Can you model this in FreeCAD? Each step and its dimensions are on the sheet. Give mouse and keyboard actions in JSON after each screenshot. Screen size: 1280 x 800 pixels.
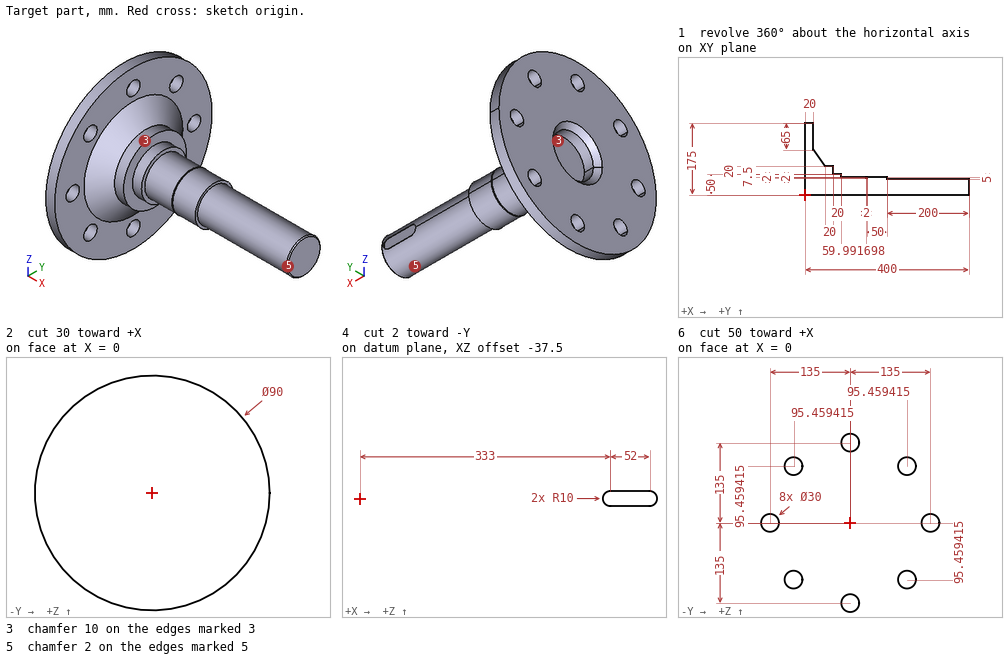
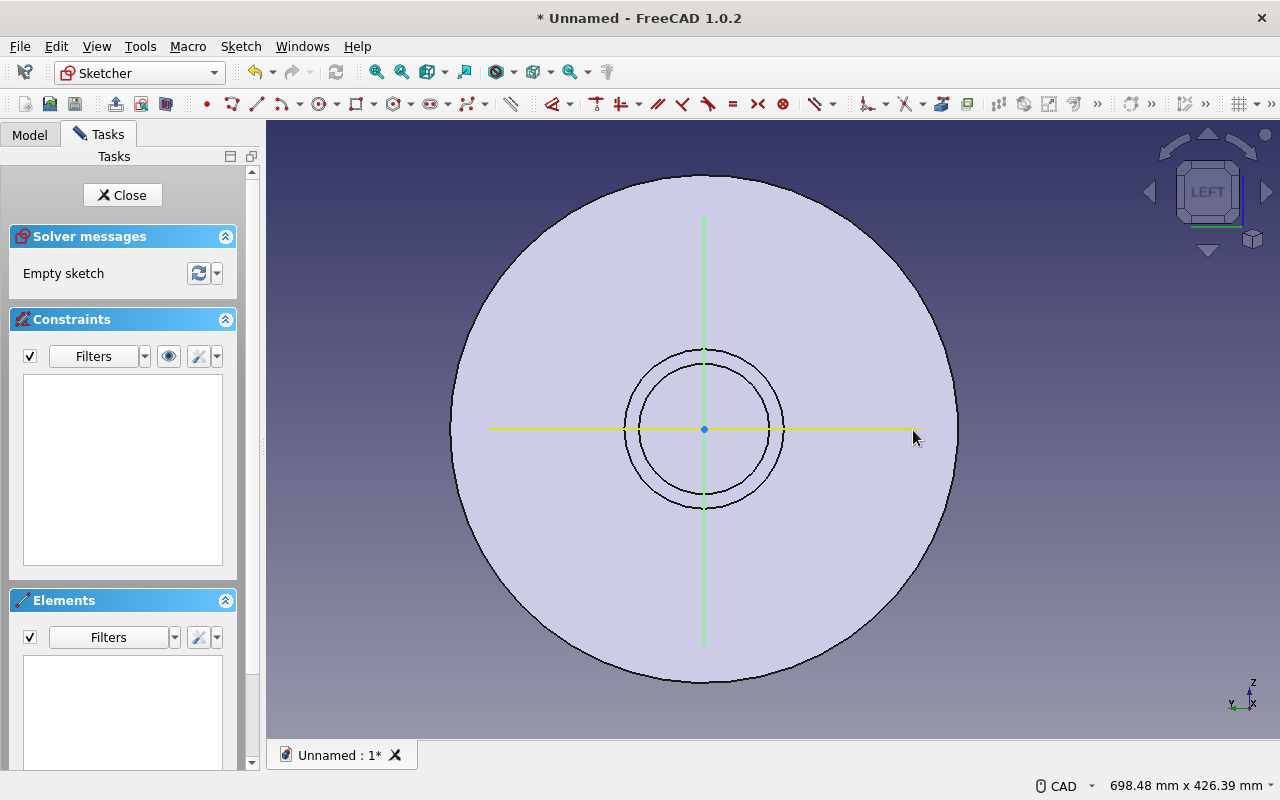
{"action": "left_click", "coordinate": [318, 104]}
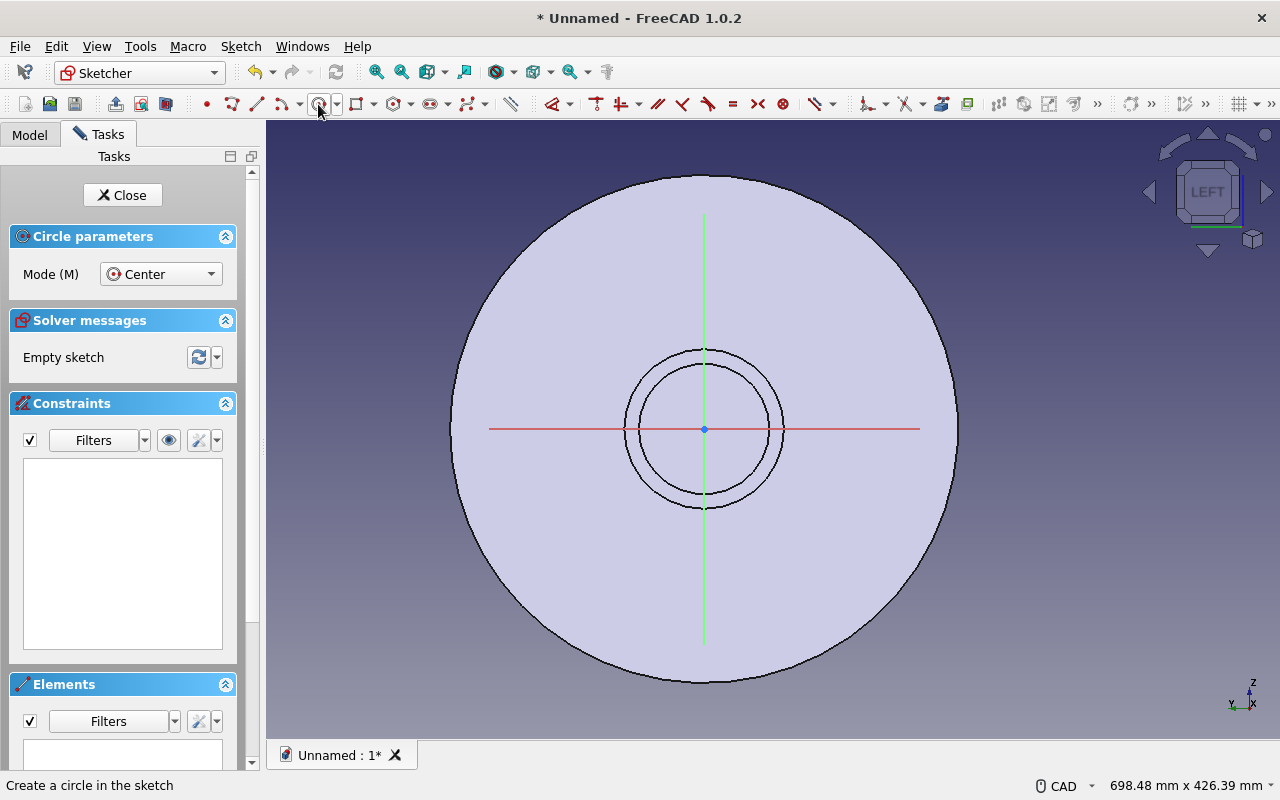
{"action": "left_click", "coordinate": [508, 429]}
{"action": "mouse_move", "coordinate": [524, 414]}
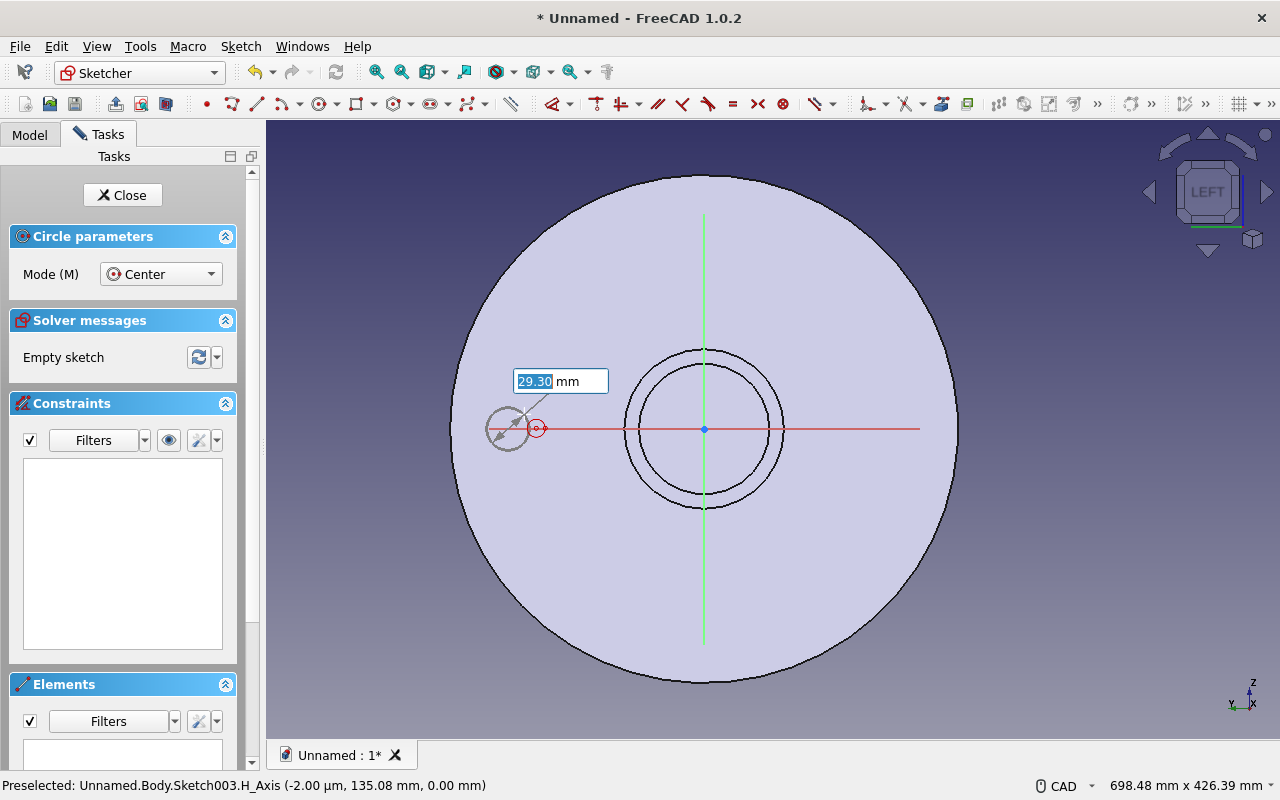
{"action": "type", "text": "30"}
{"action": "key", "text": "Return"}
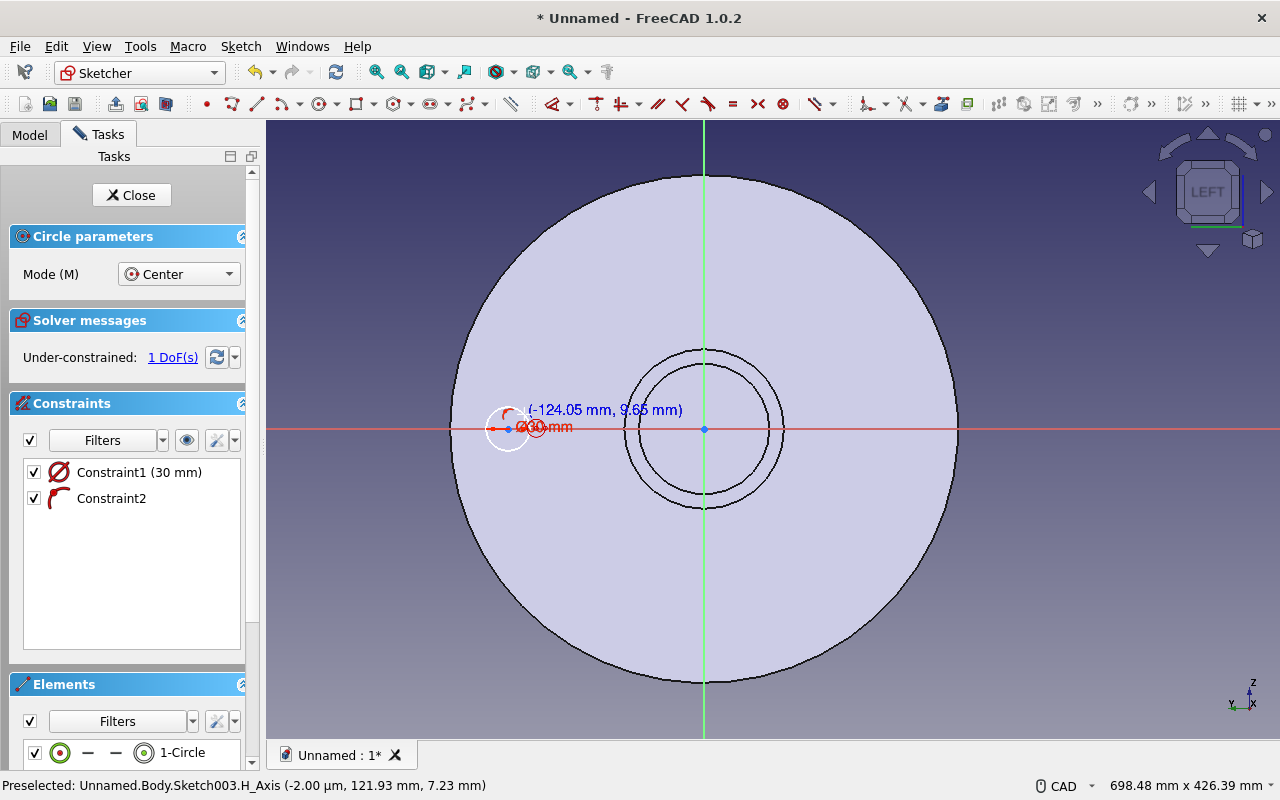
{"action": "left_click", "coordinate": [566, 290]}
{"action": "mouse_move", "coordinate": [581, 275]}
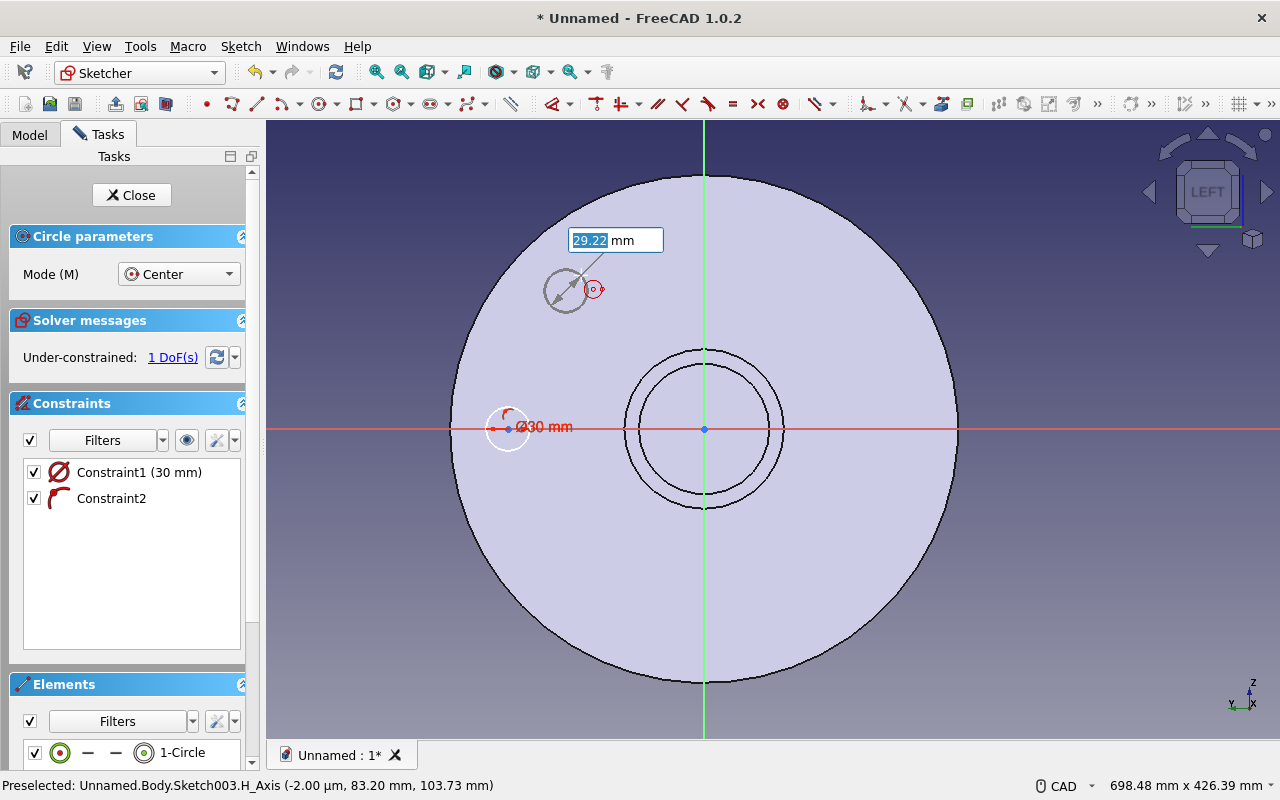
{"action": "type", "text": "30"}
{"action": "key", "text": "Return"}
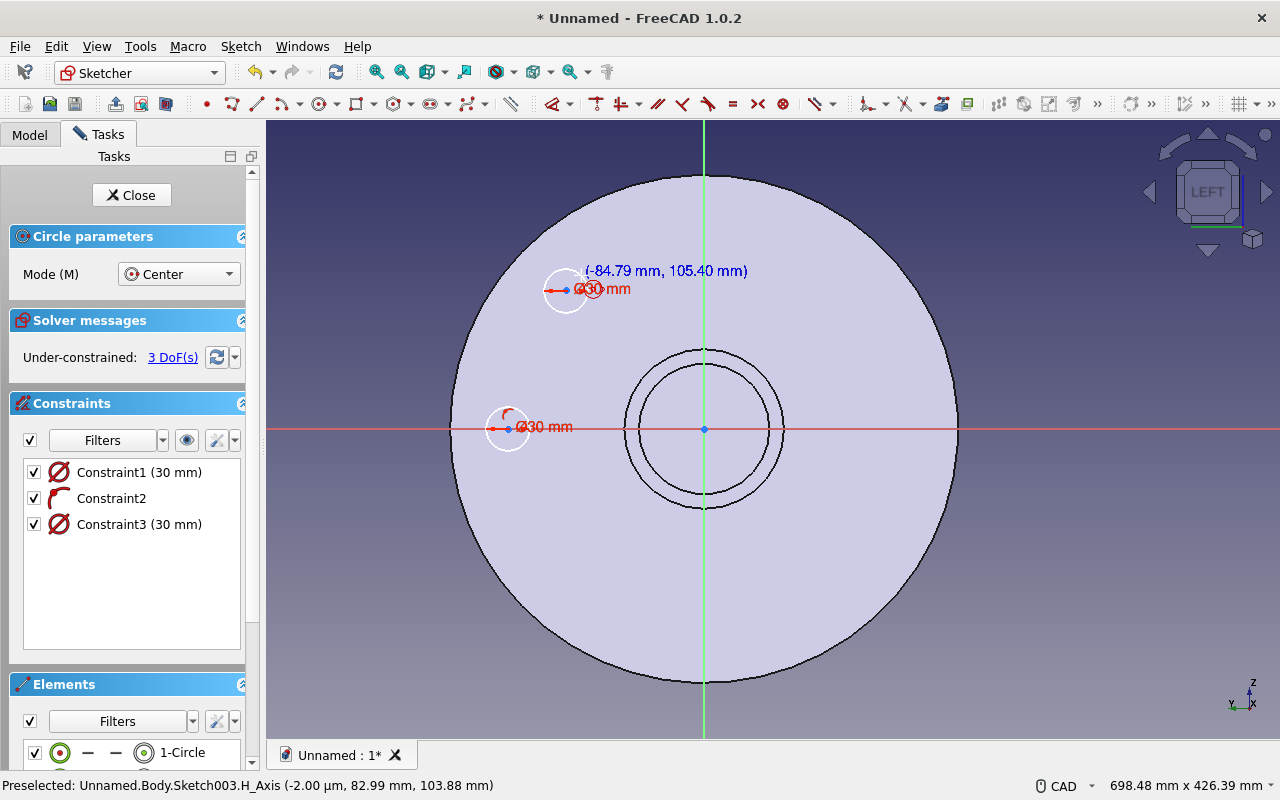
{"action": "left_click", "coordinate": [704, 233]}
{"action": "mouse_move", "coordinate": [719, 218]}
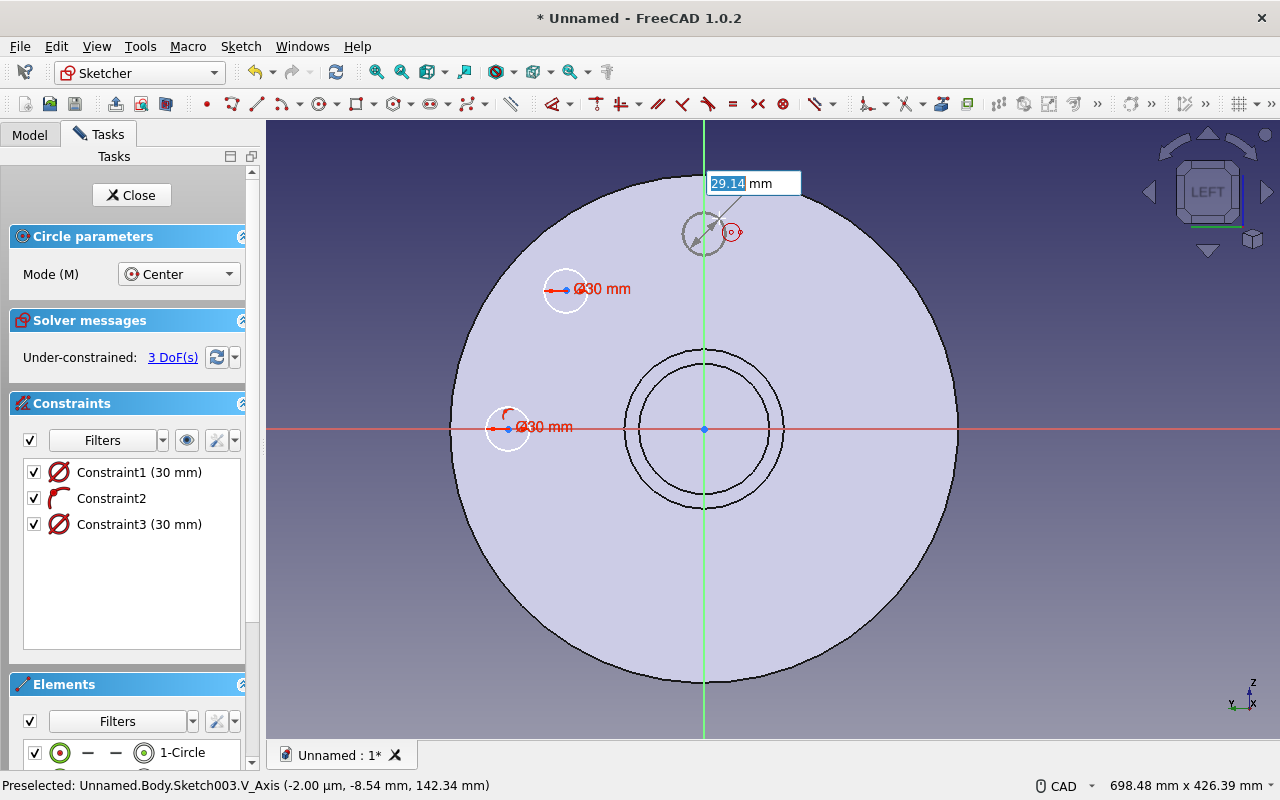
{"action": "type", "text": "30"}
{"action": "key", "text": "Return"}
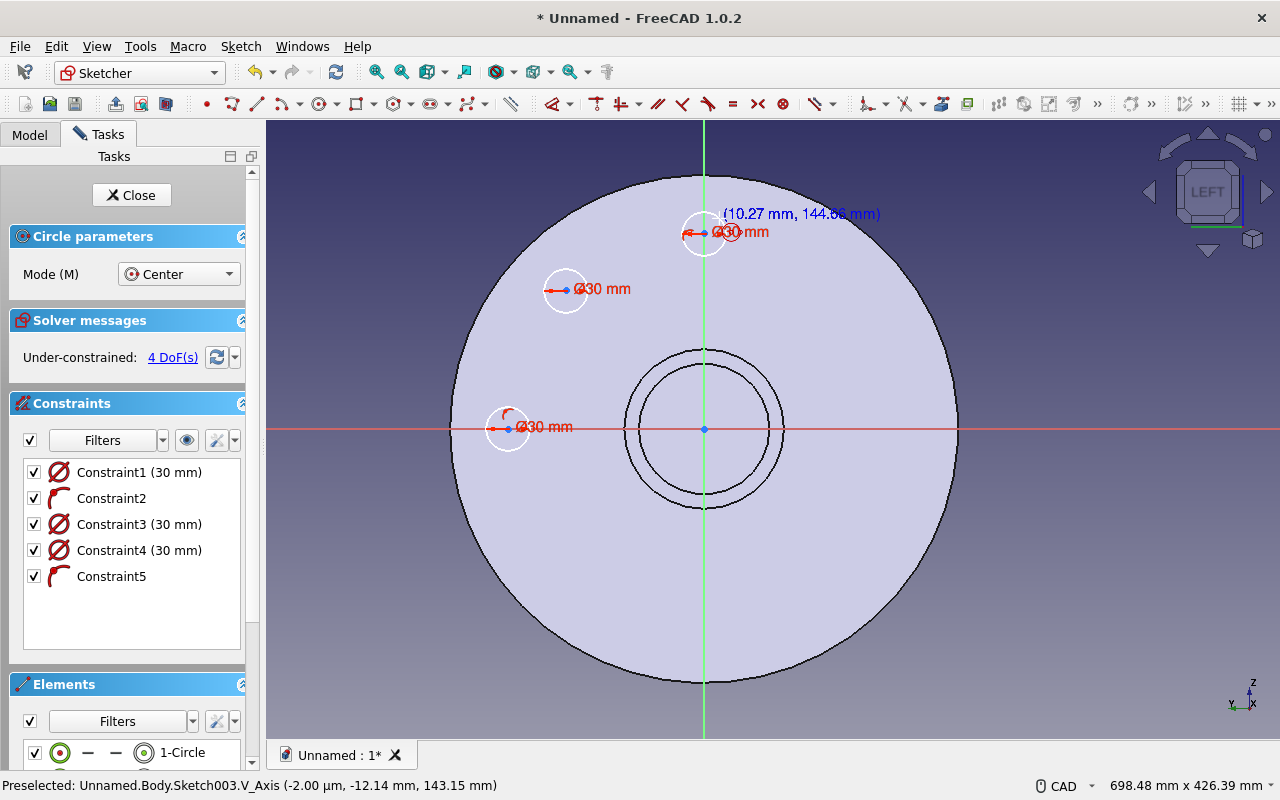
{"action": "left_click", "coordinate": [843, 290]}
{"action": "mouse_move", "coordinate": [858, 275]}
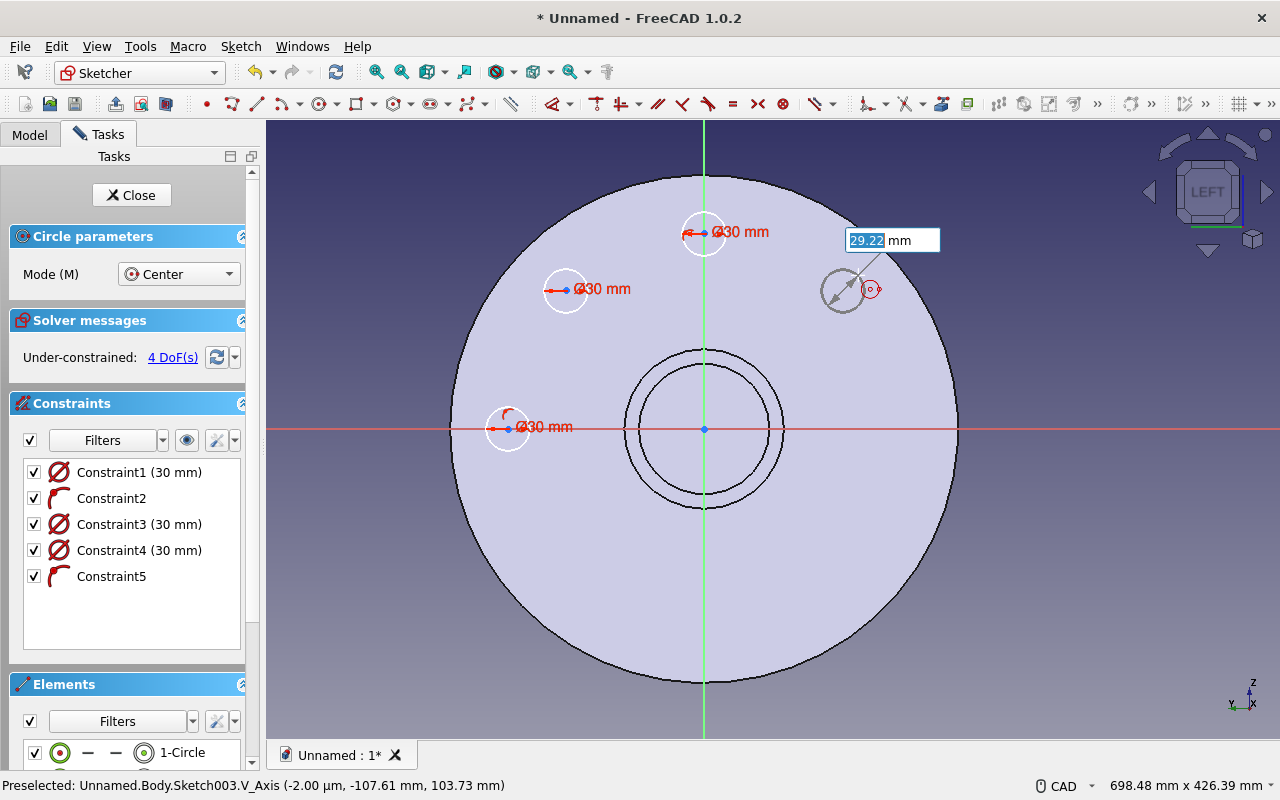
{"action": "type", "text": "30"}
{"action": "key", "text": "Return"}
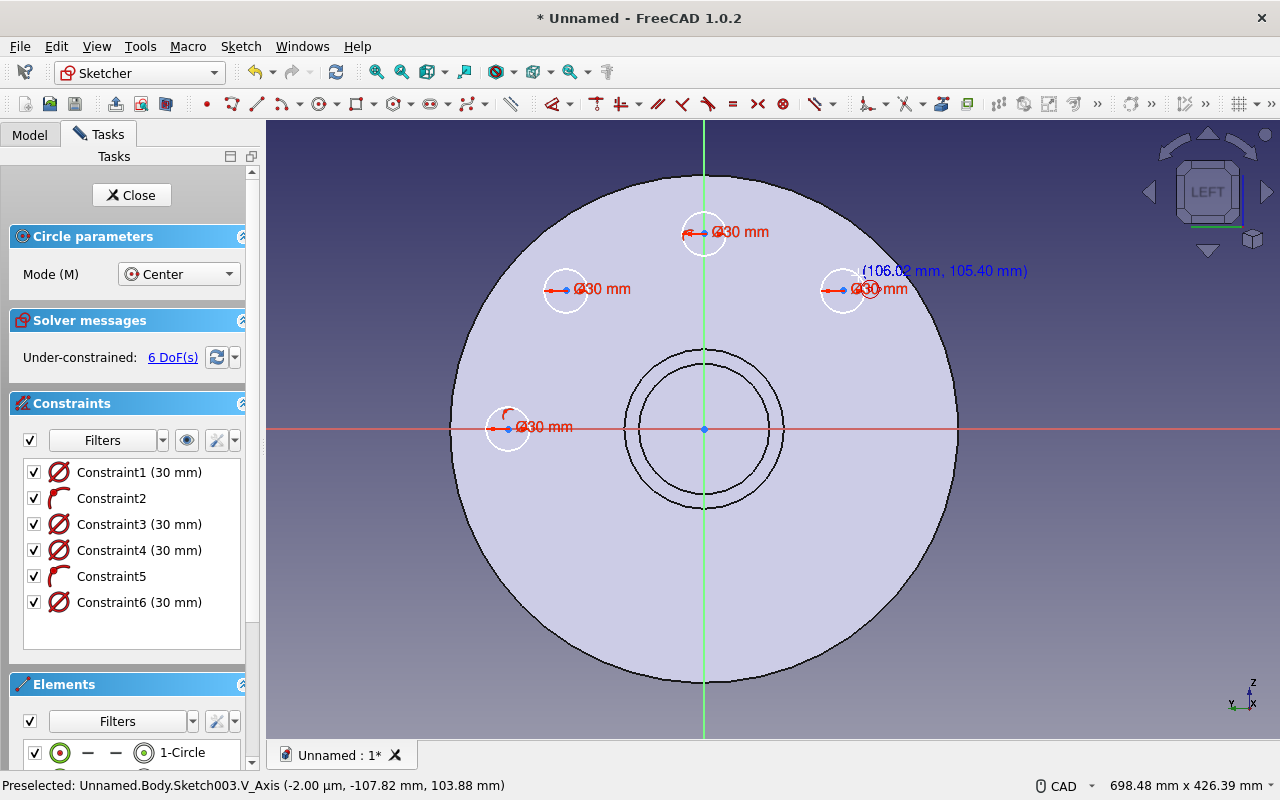
{"action": "left_click", "coordinate": [900, 429]}
{"action": "mouse_move", "coordinate": [915, 414]}